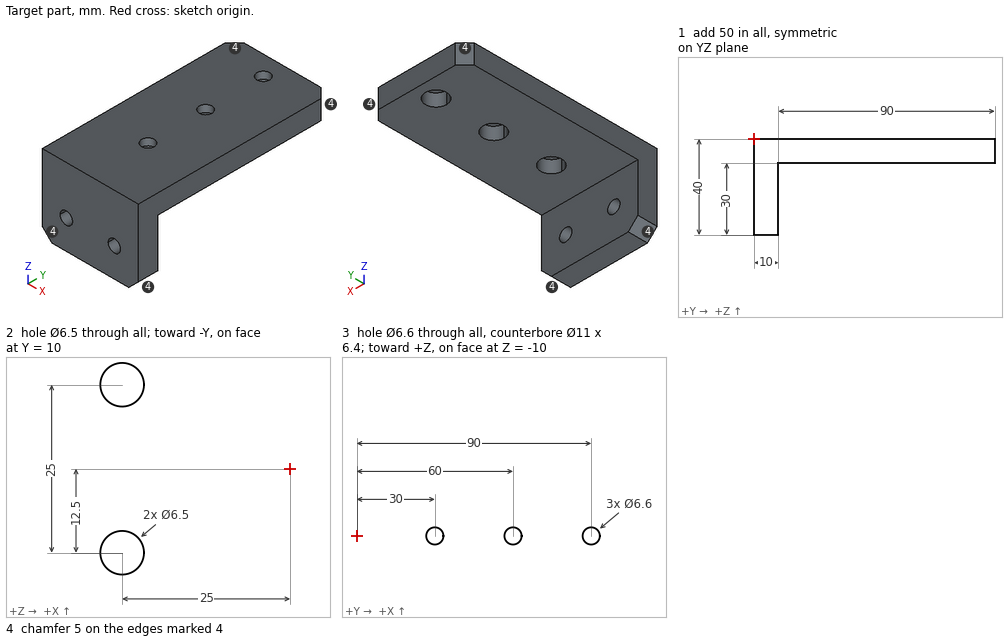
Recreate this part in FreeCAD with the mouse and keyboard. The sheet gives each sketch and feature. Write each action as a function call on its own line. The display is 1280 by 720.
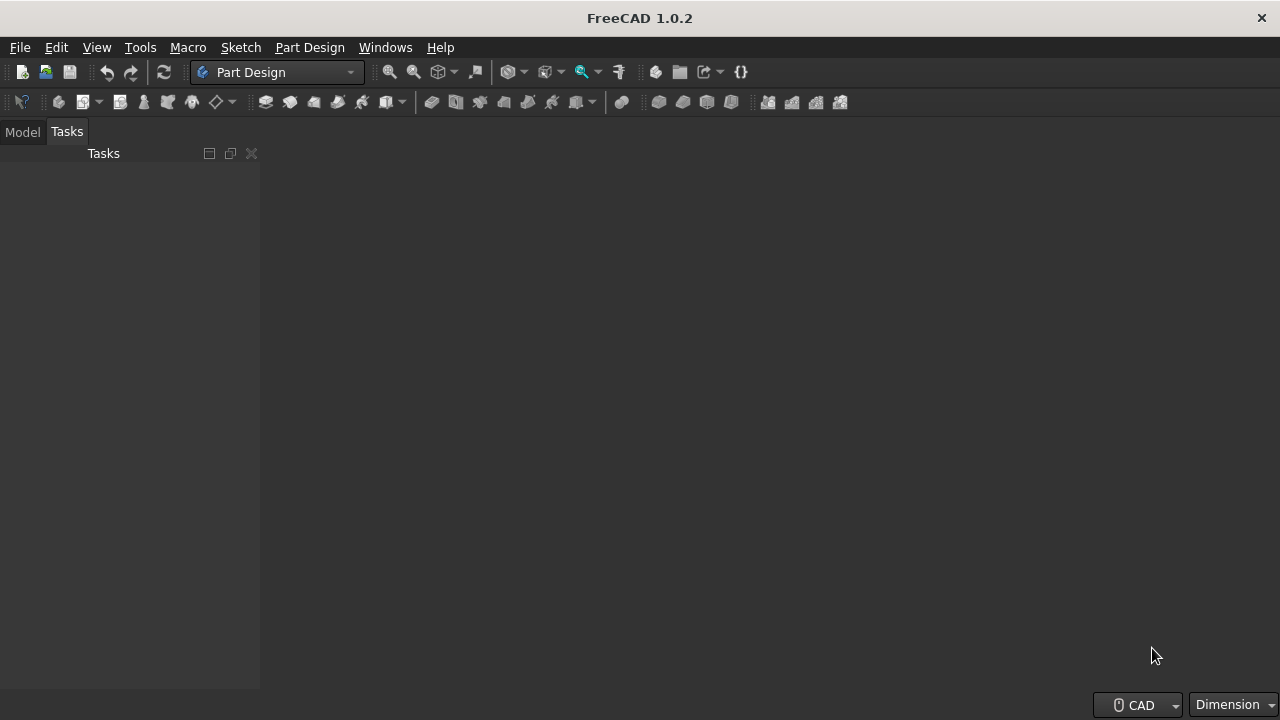
click(22, 72)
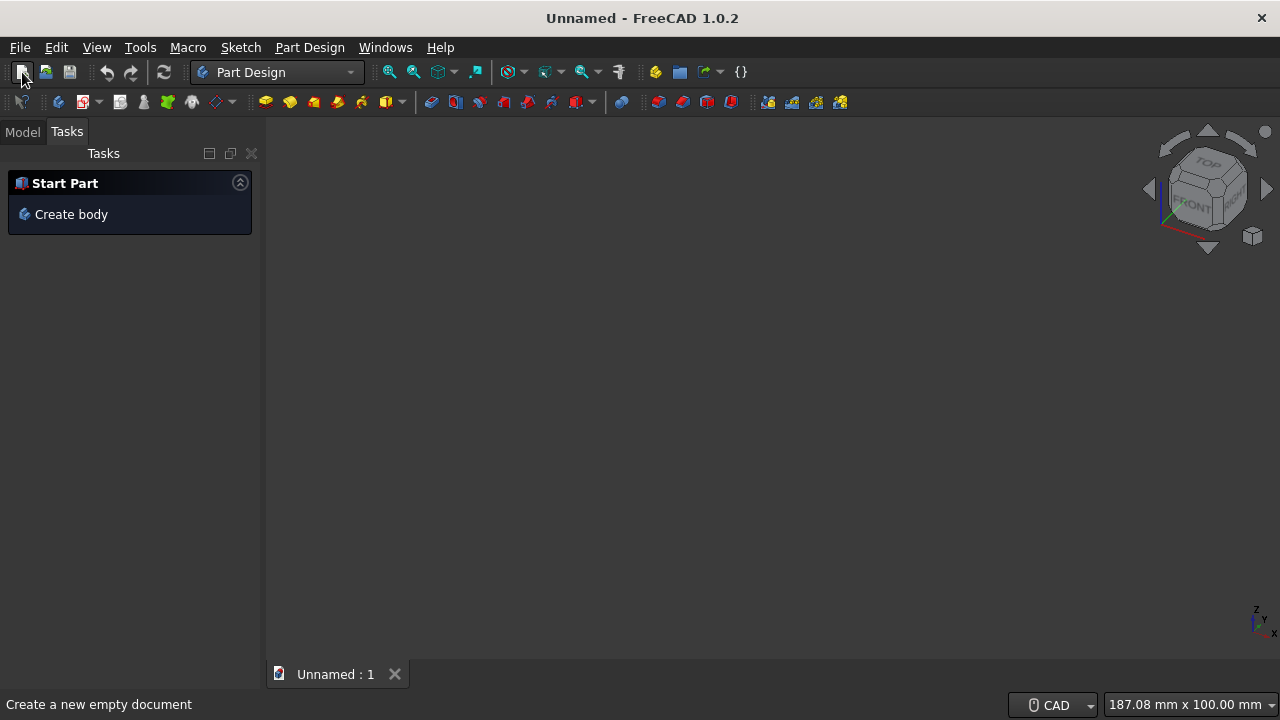
click(84, 102)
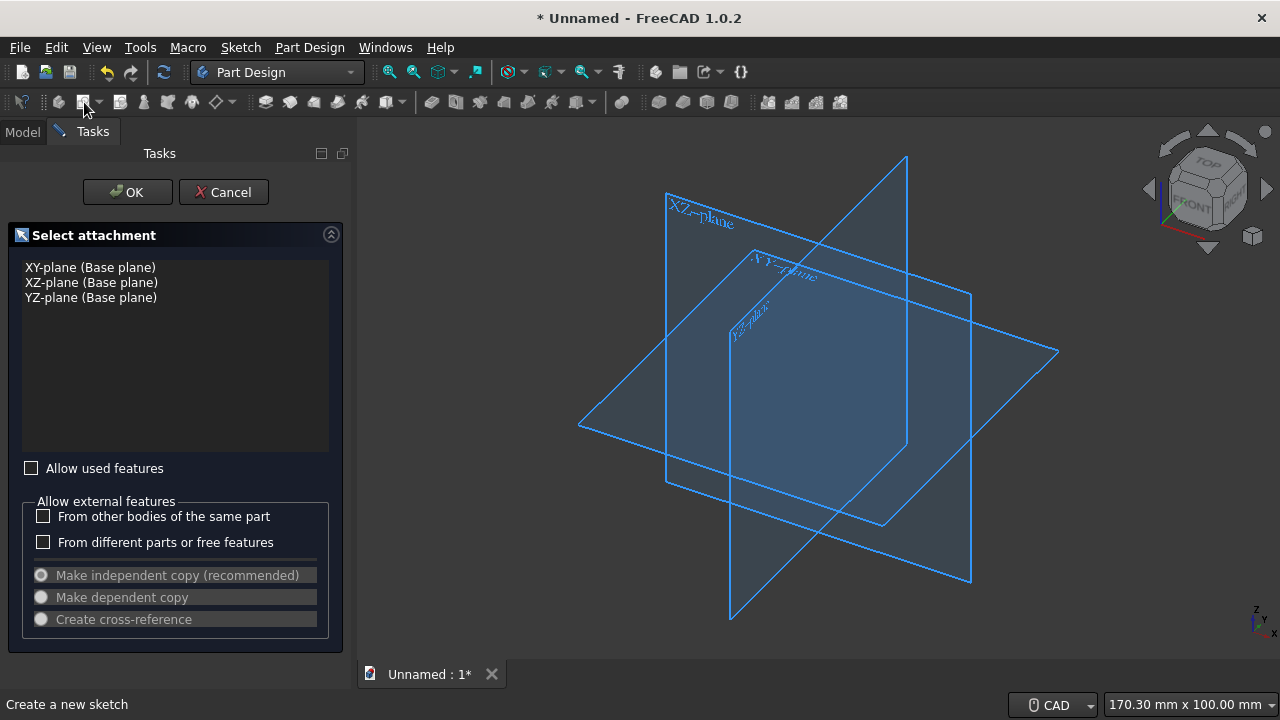
click(82, 298)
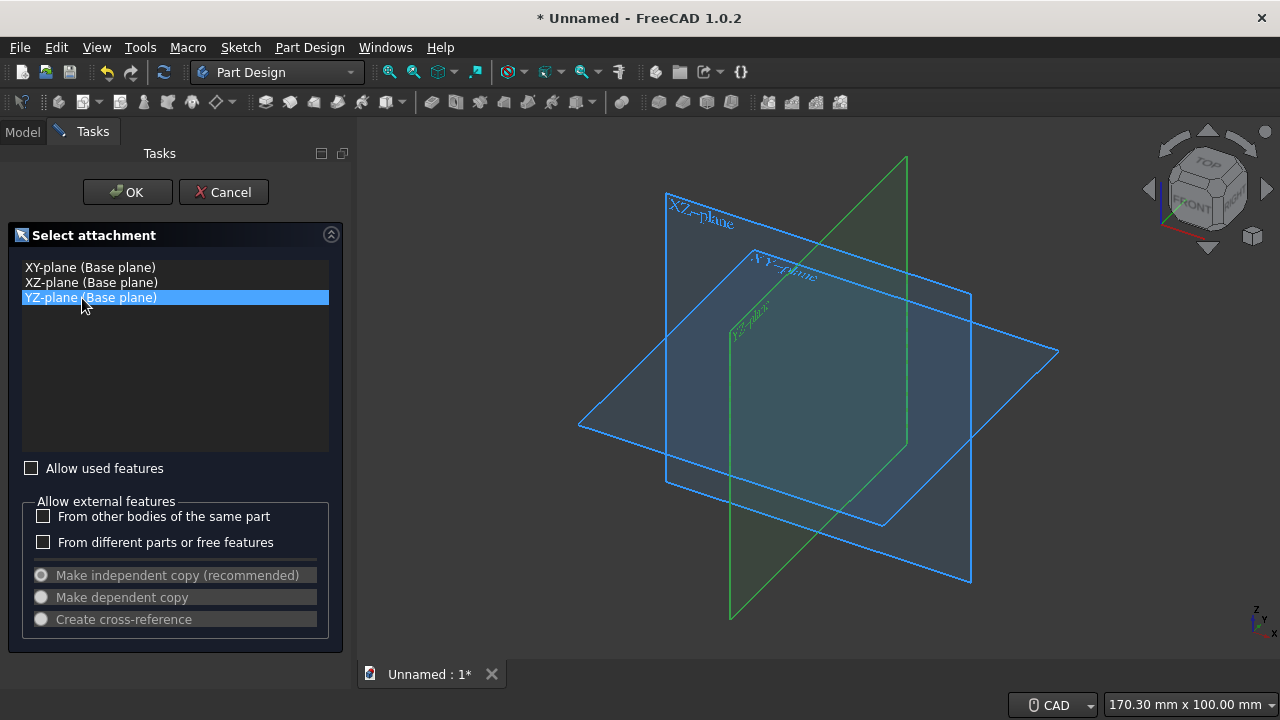
click(128, 192)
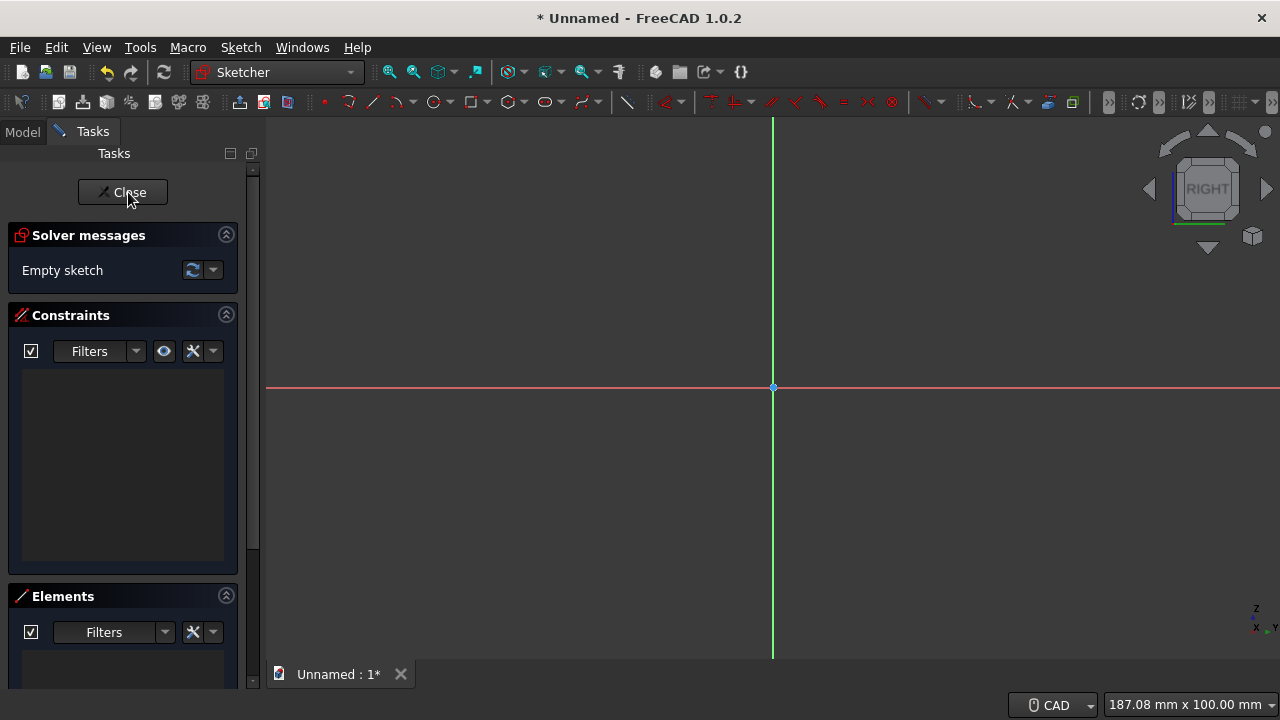
scroll(294, 168, down, 2)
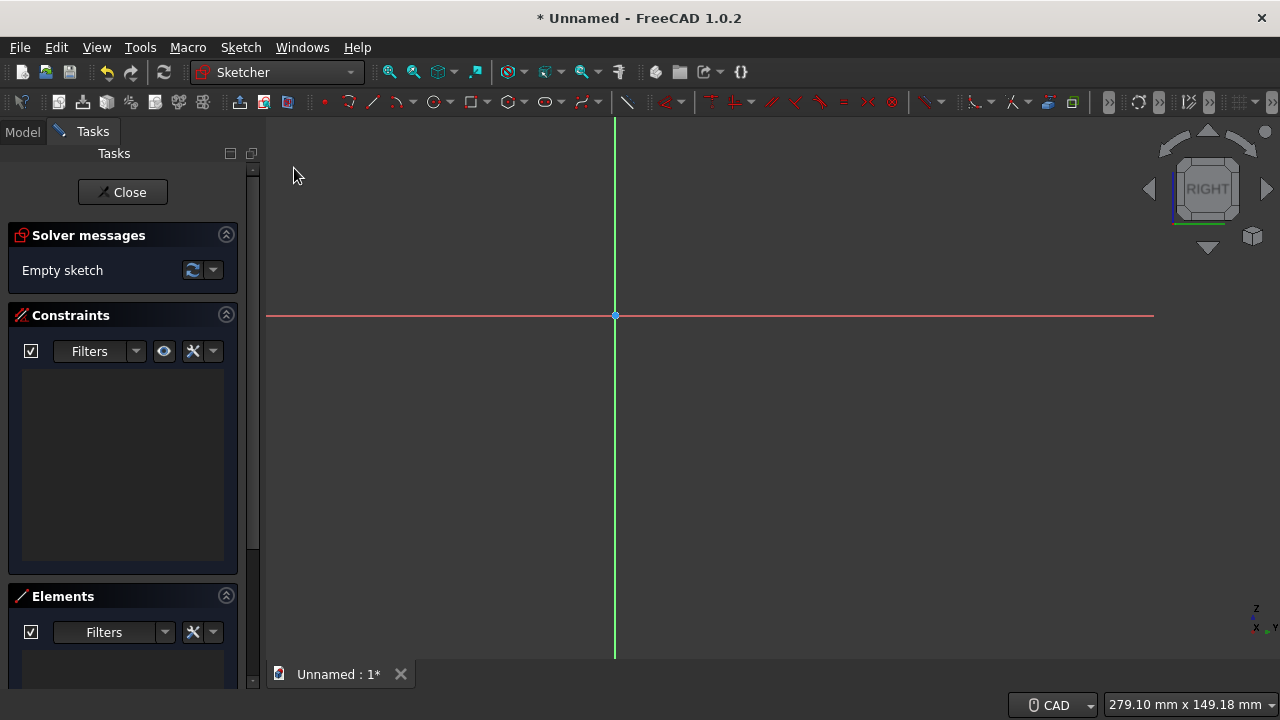
scroll(984, 388, up, 2)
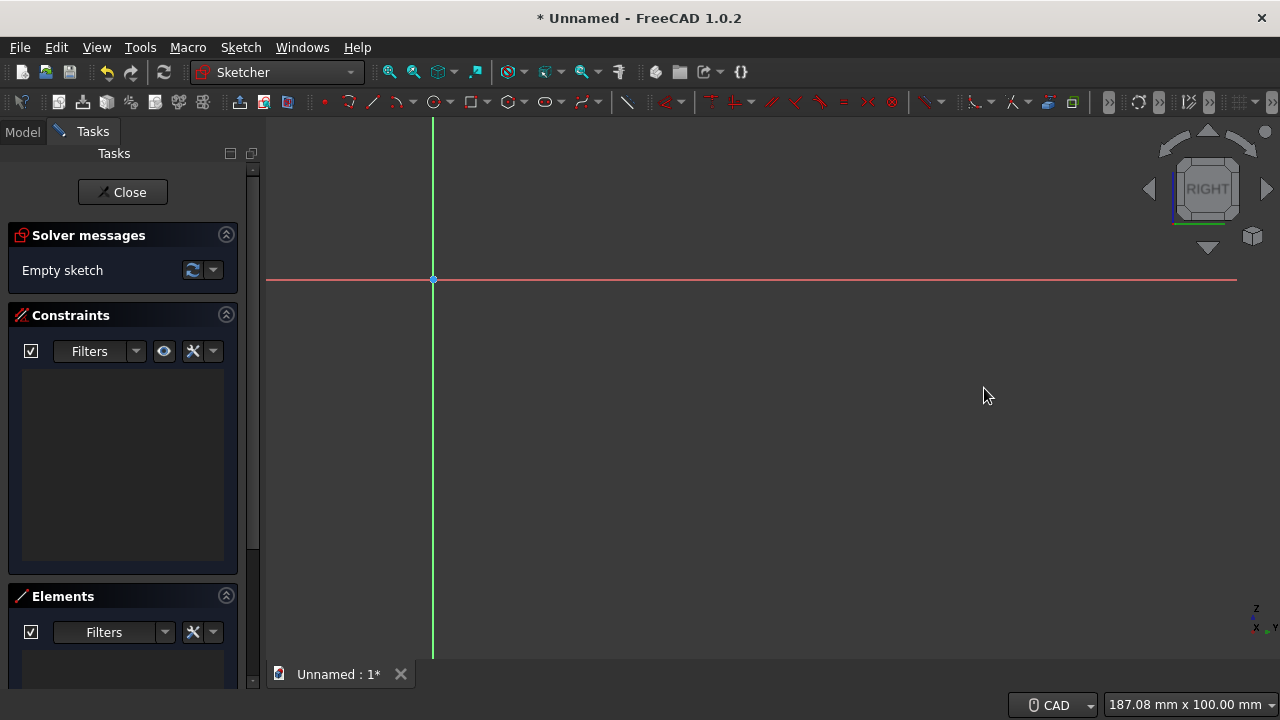
click(350, 102)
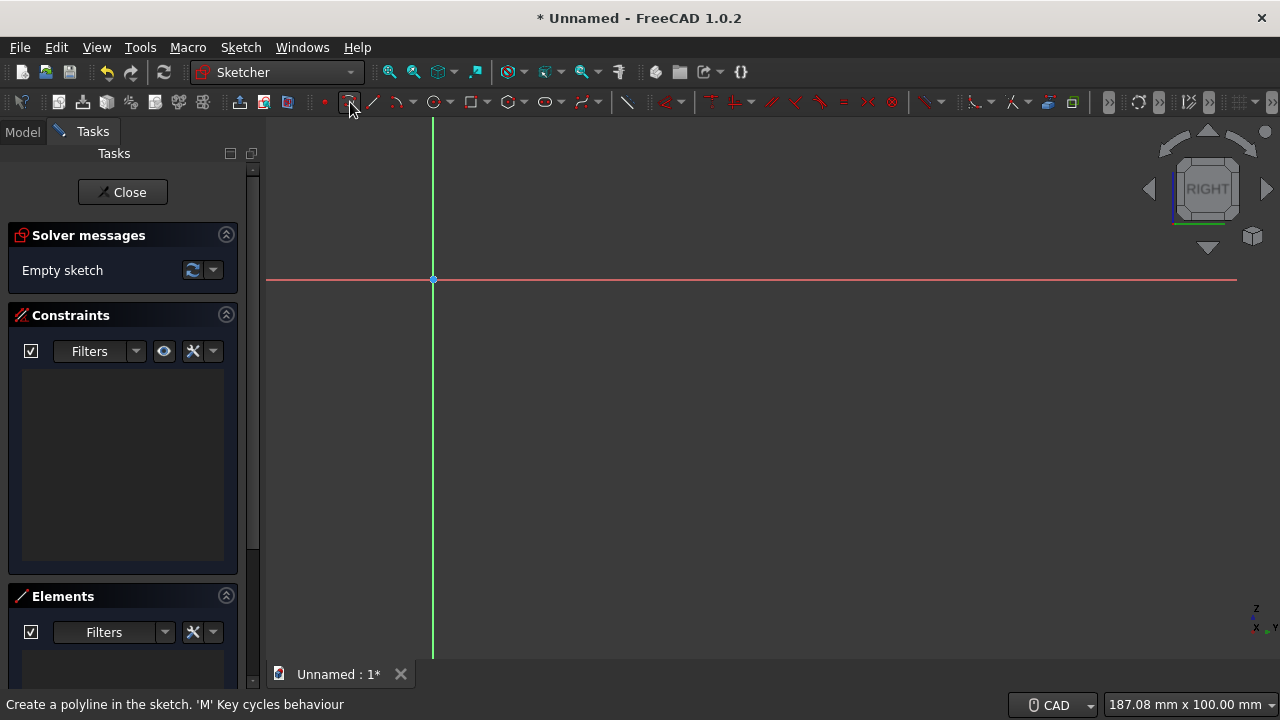
click(433, 280)
click(442, 496)
click(488, 496)
click(488, 334)
click(975, 334)
click(975, 289)
click(433, 280)
key(Escape)
key(Escape)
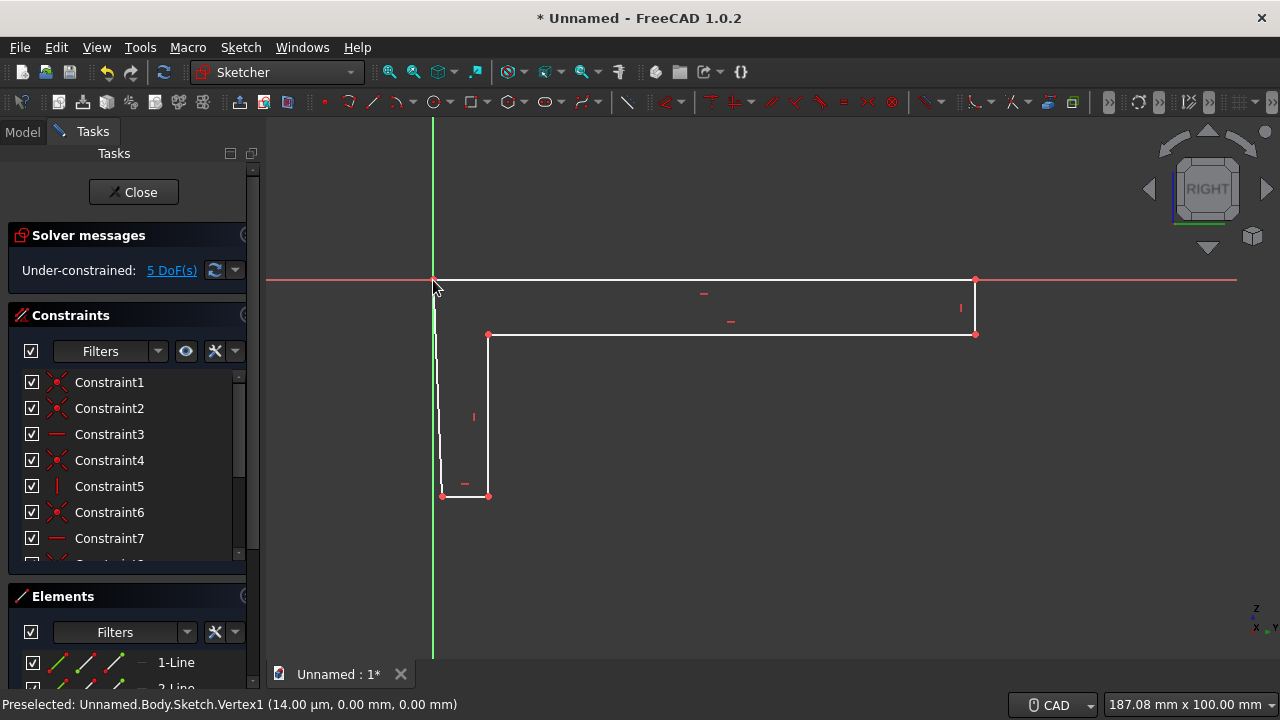
click(436, 345)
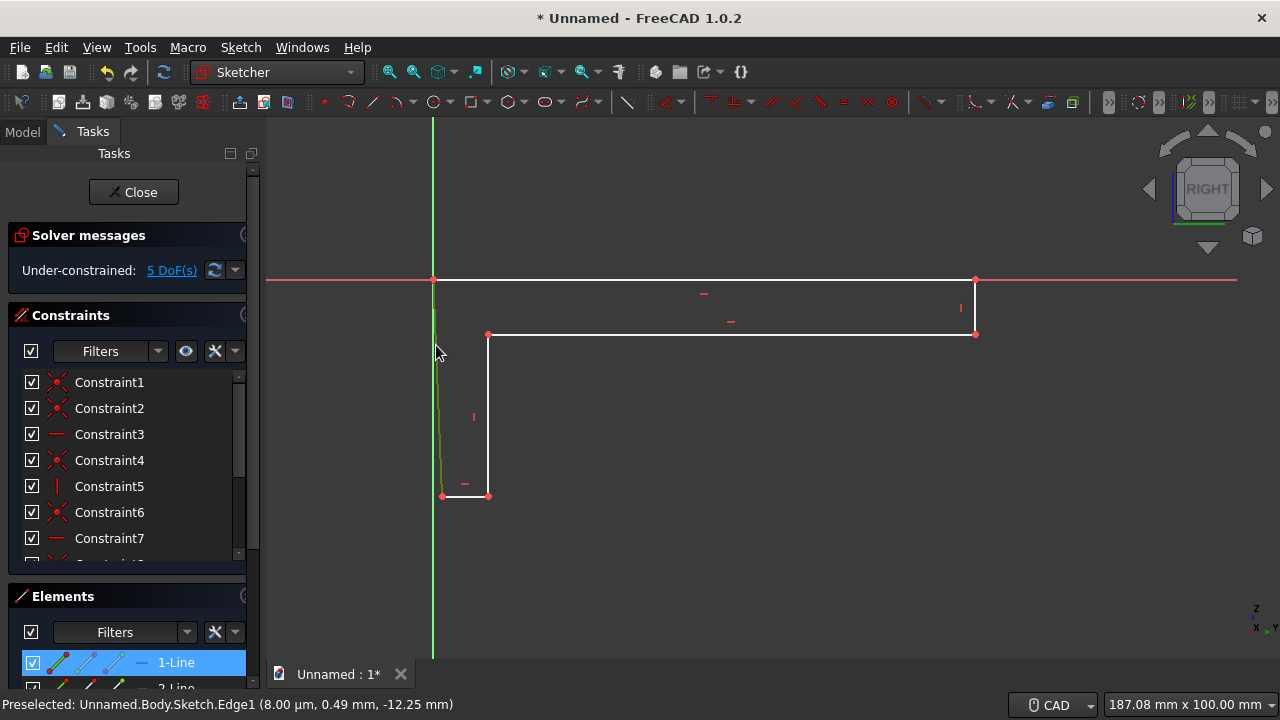
click(754, 102)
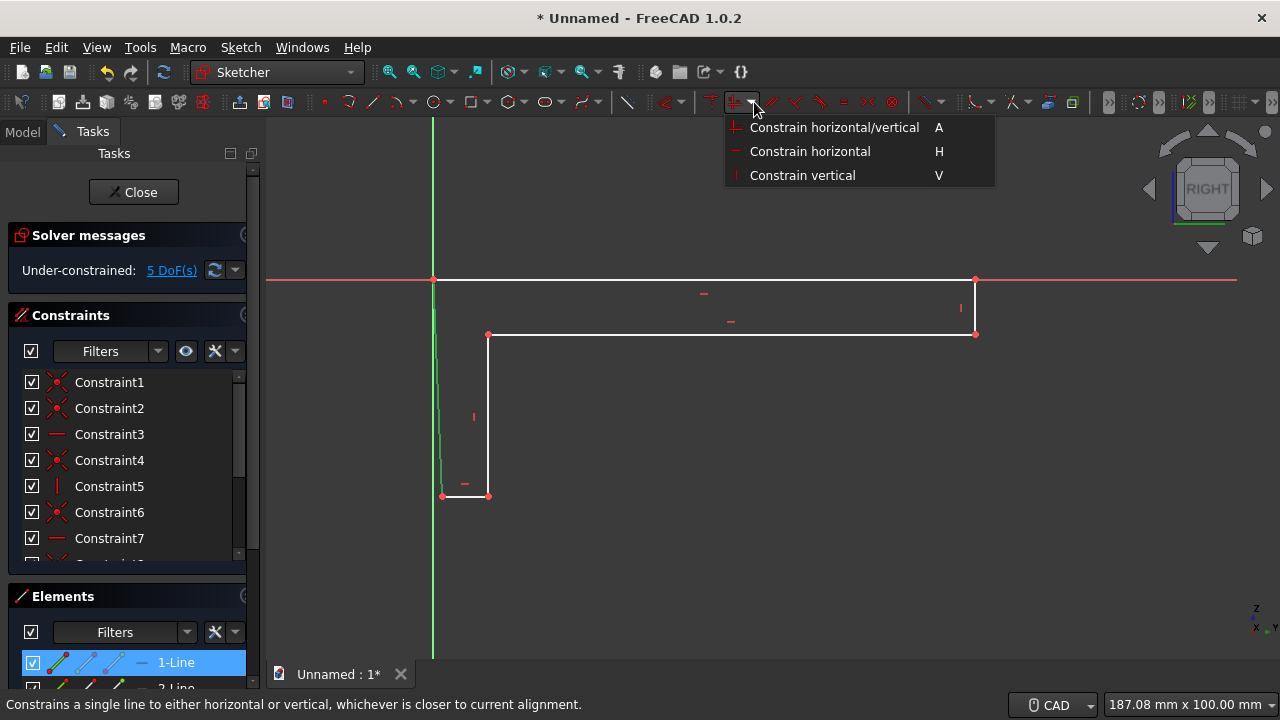
click(860, 175)